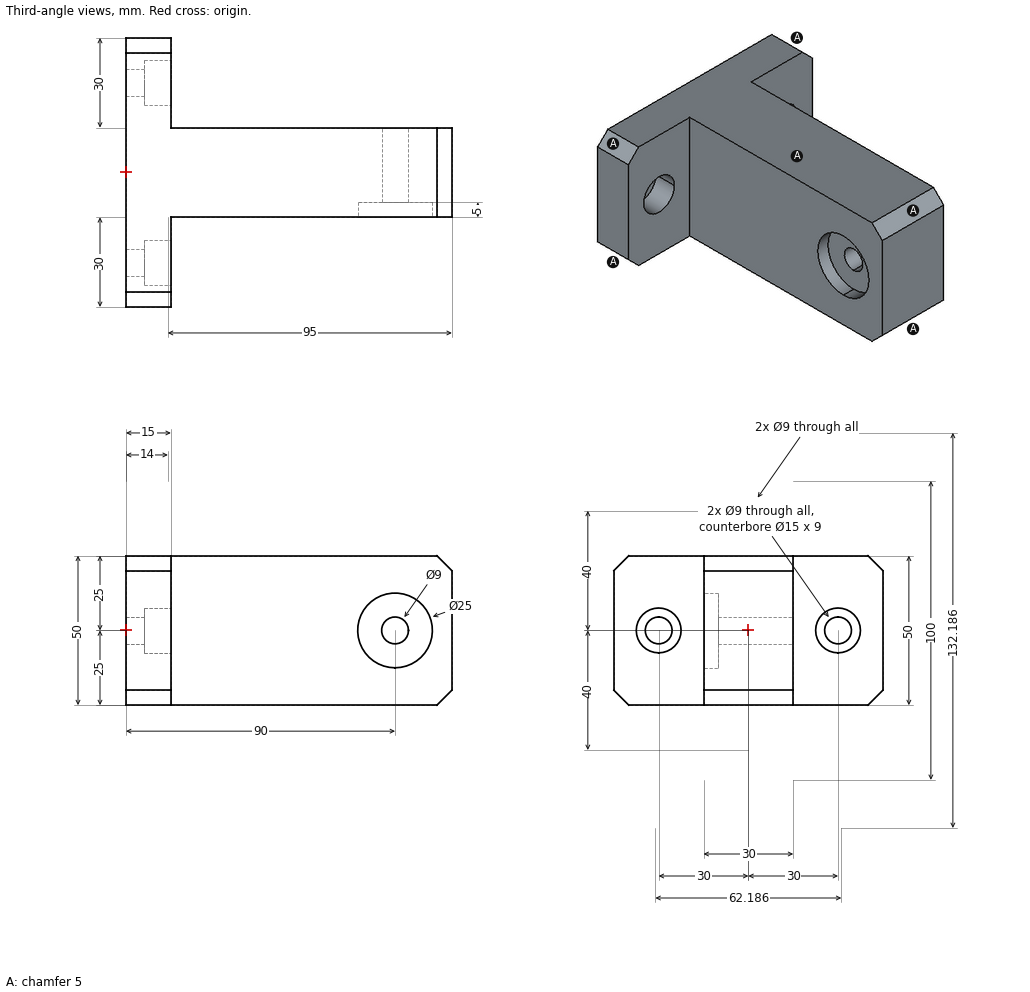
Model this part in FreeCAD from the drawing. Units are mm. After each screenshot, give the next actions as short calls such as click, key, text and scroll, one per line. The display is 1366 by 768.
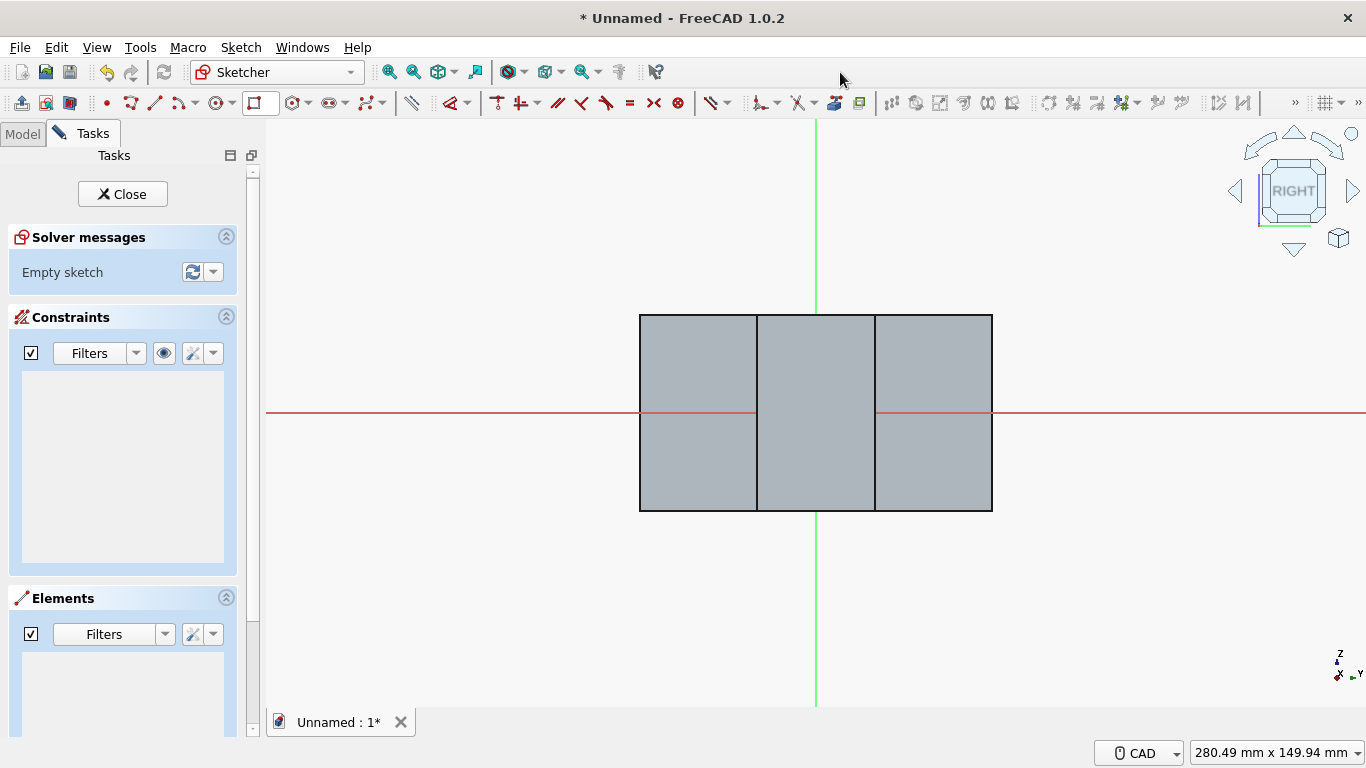
click(70, 104)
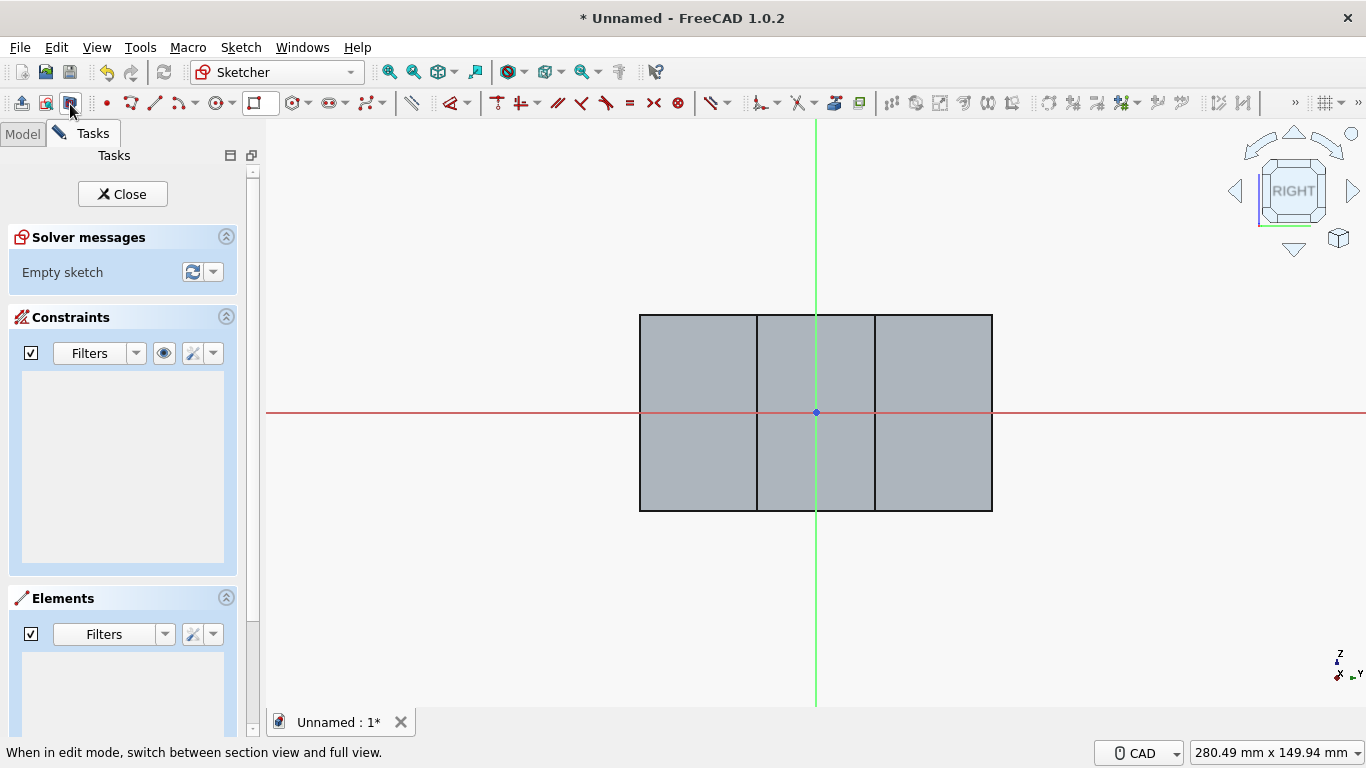
scroll(872, 413, up, 4)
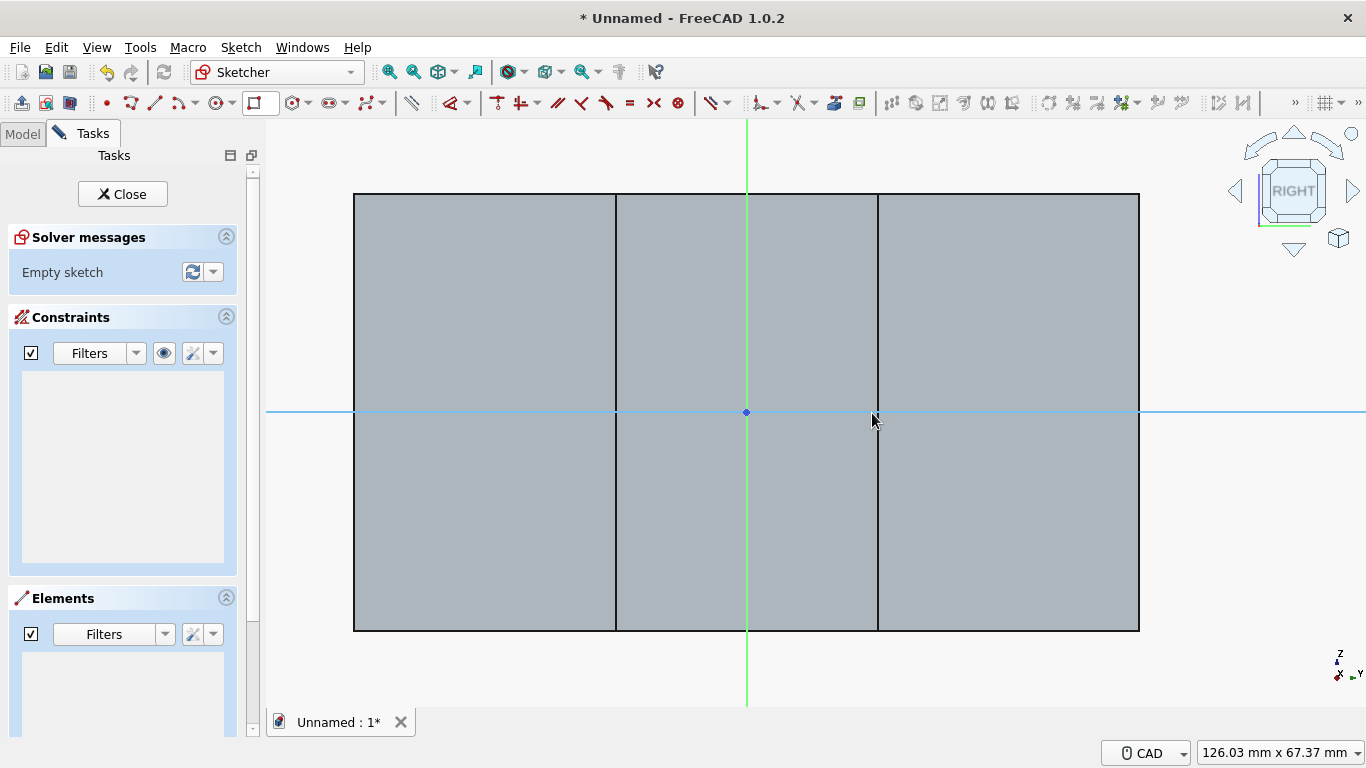
click(216, 104)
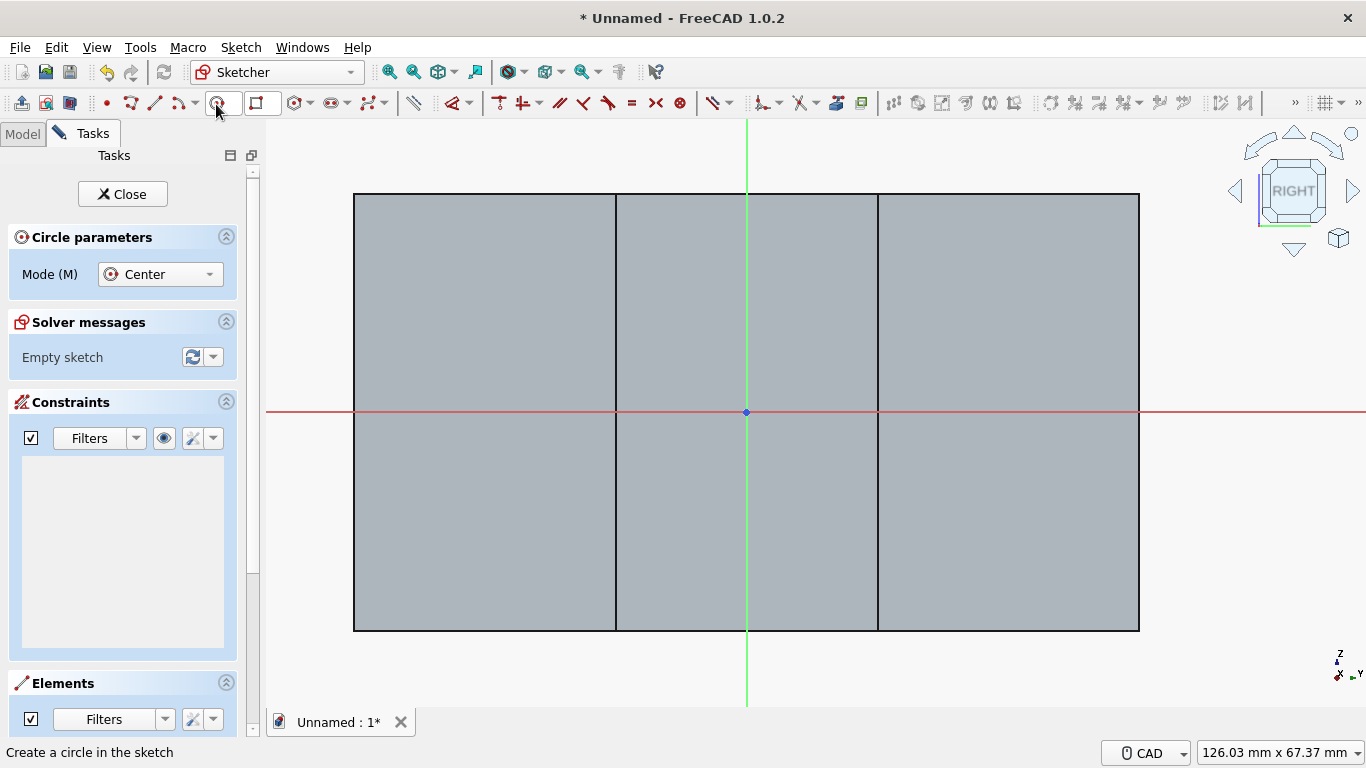
click(1009, 412)
move(1036, 385)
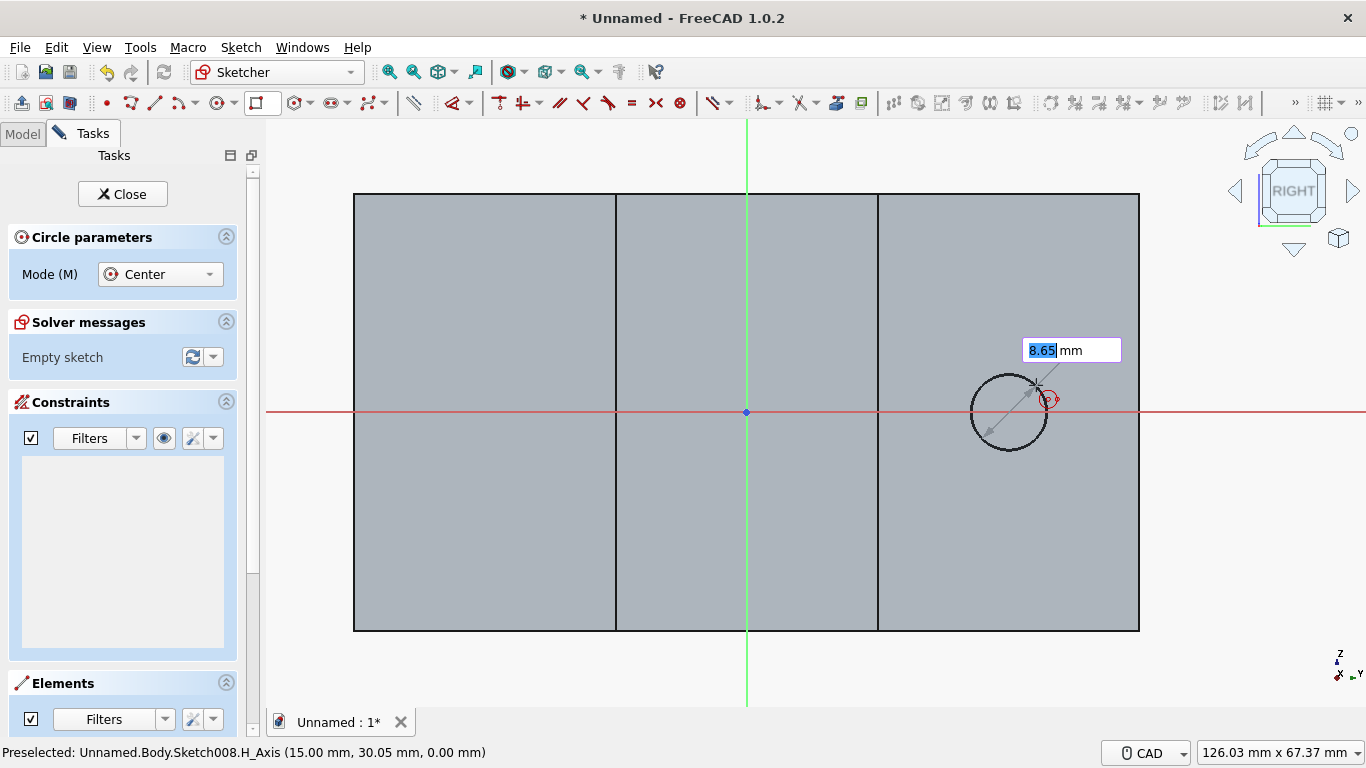
text(9)
key(Return)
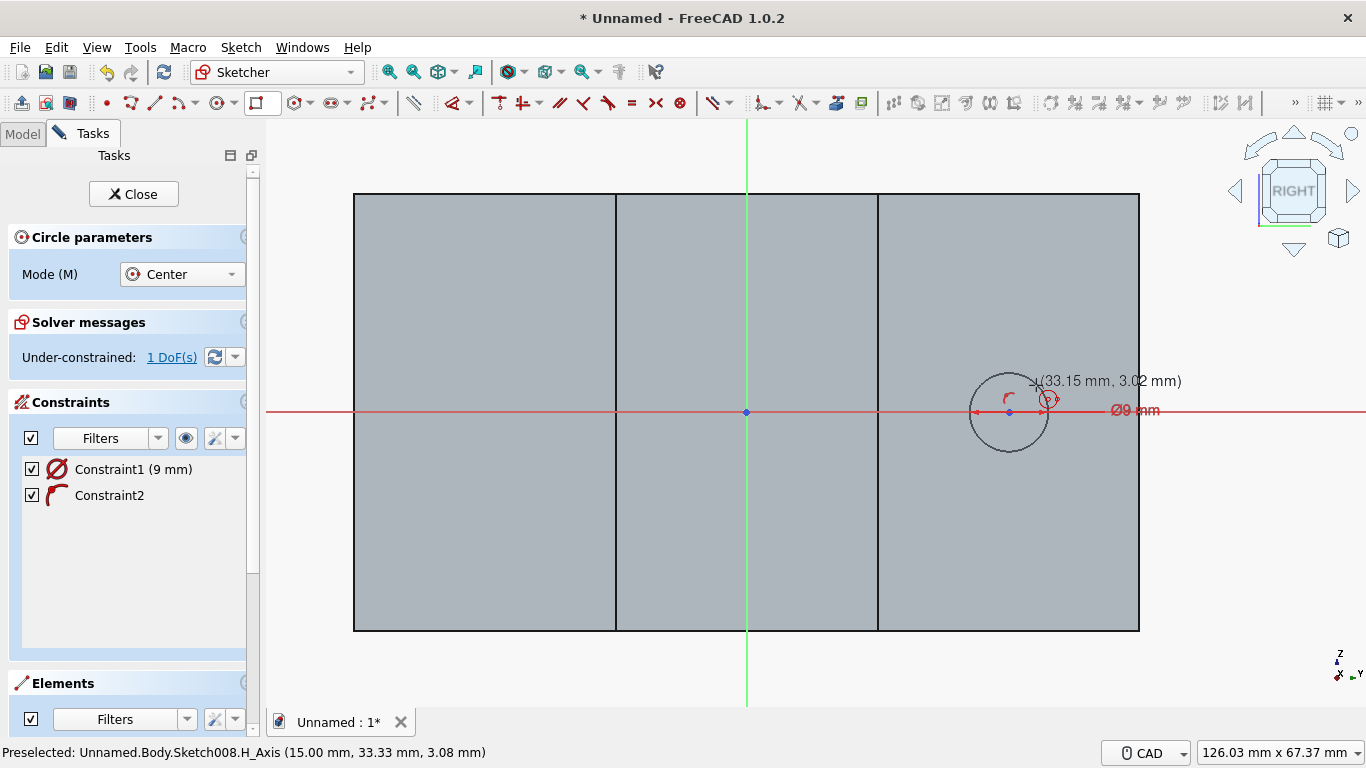
click(485, 412)
move(513, 385)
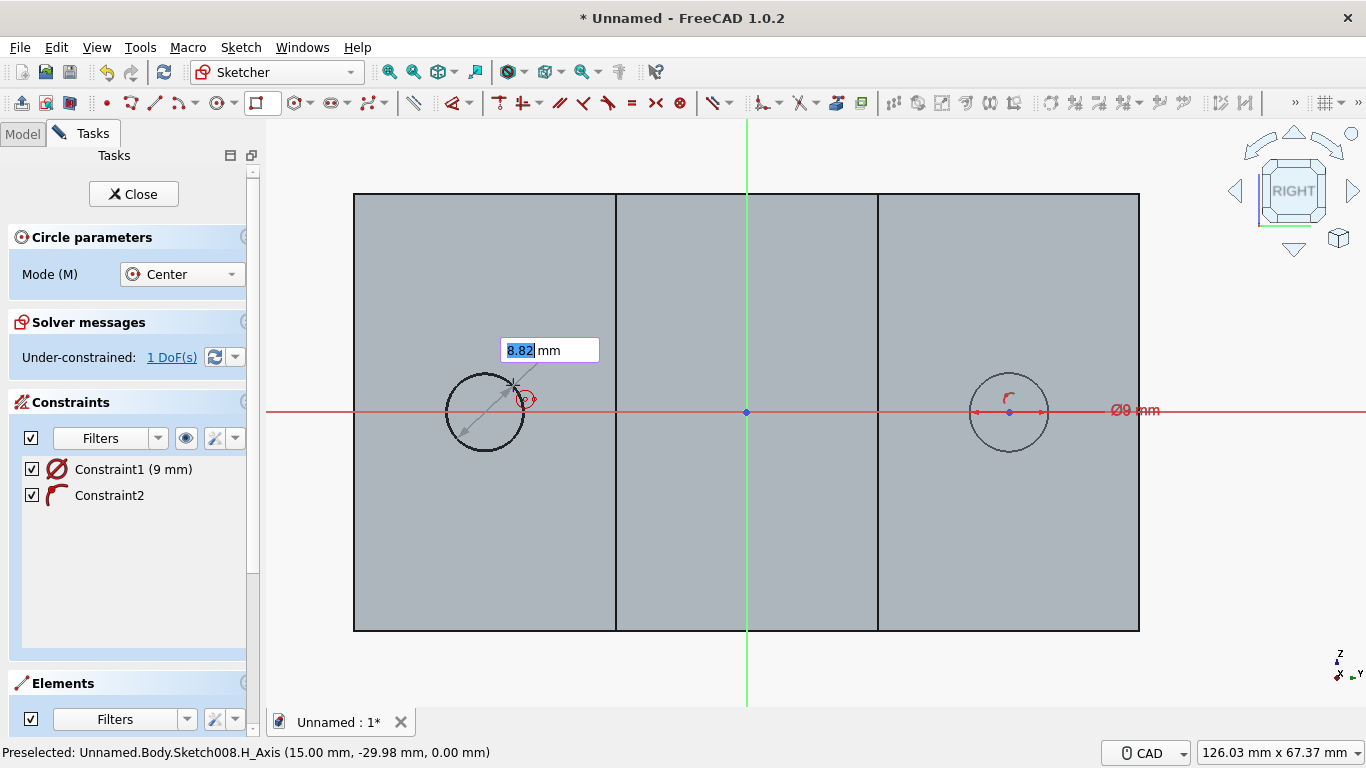
text(9)
key(Return)
key(Escape)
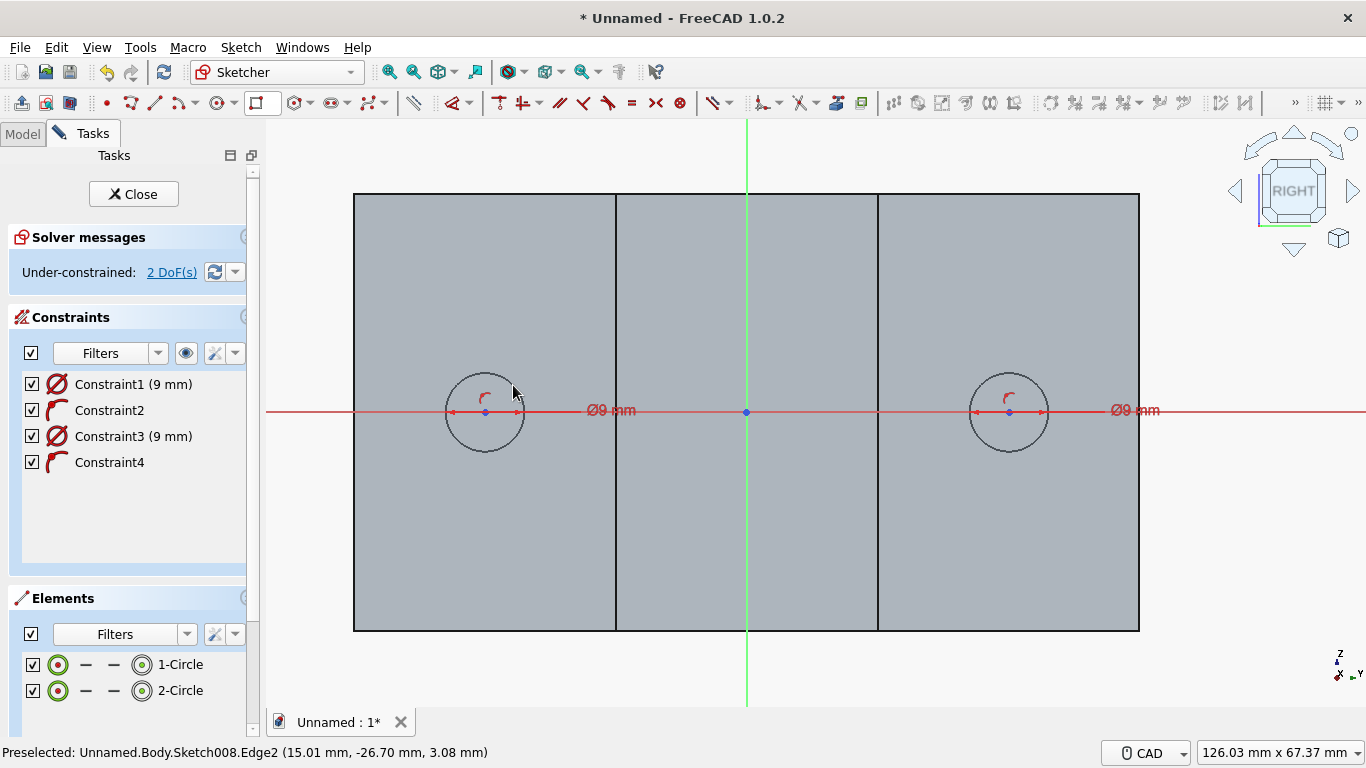
click(452, 104)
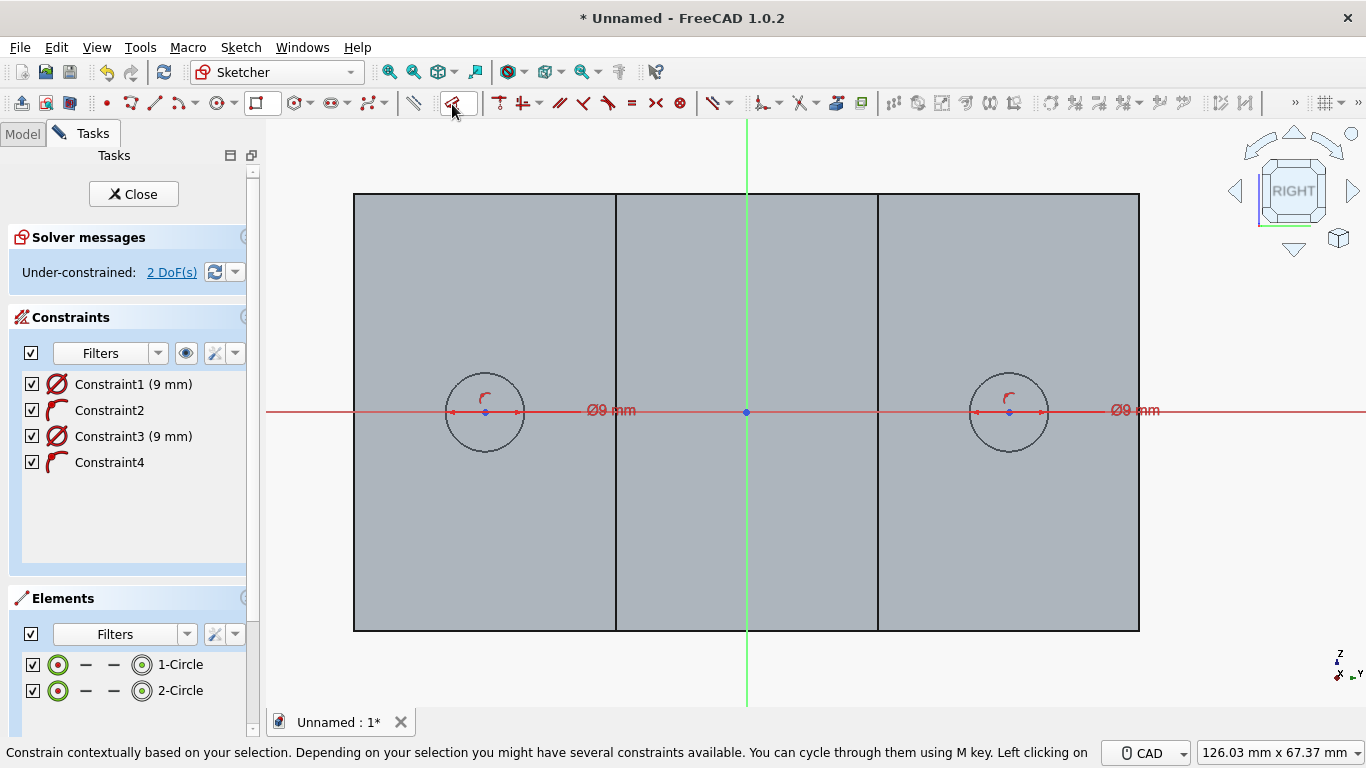
click(1009, 412)
click(878, 446)